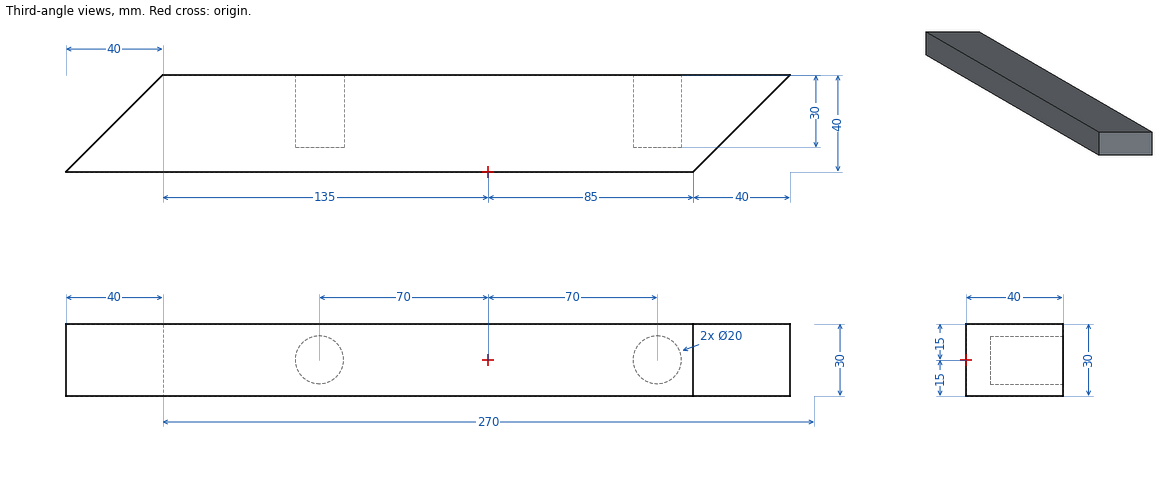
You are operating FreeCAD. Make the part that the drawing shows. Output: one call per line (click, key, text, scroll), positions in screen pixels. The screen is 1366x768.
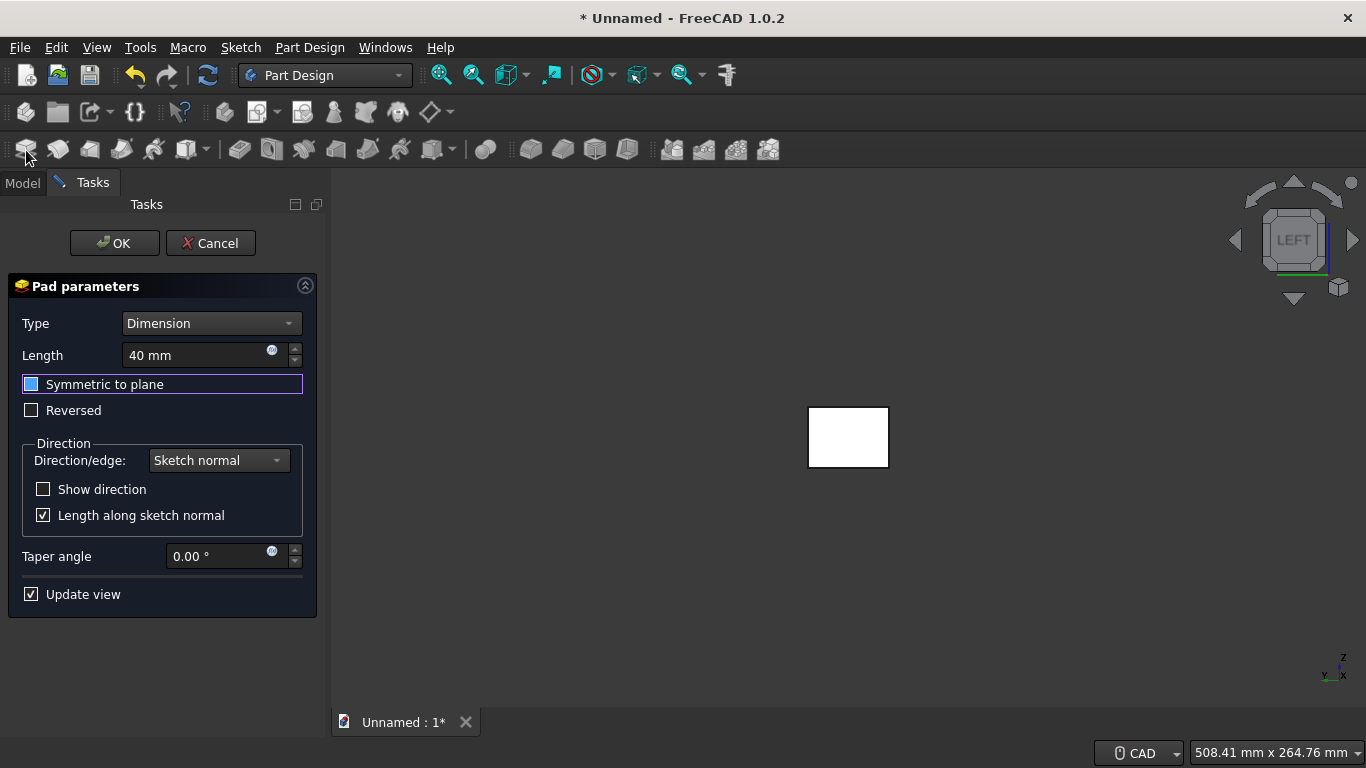
click(115, 243)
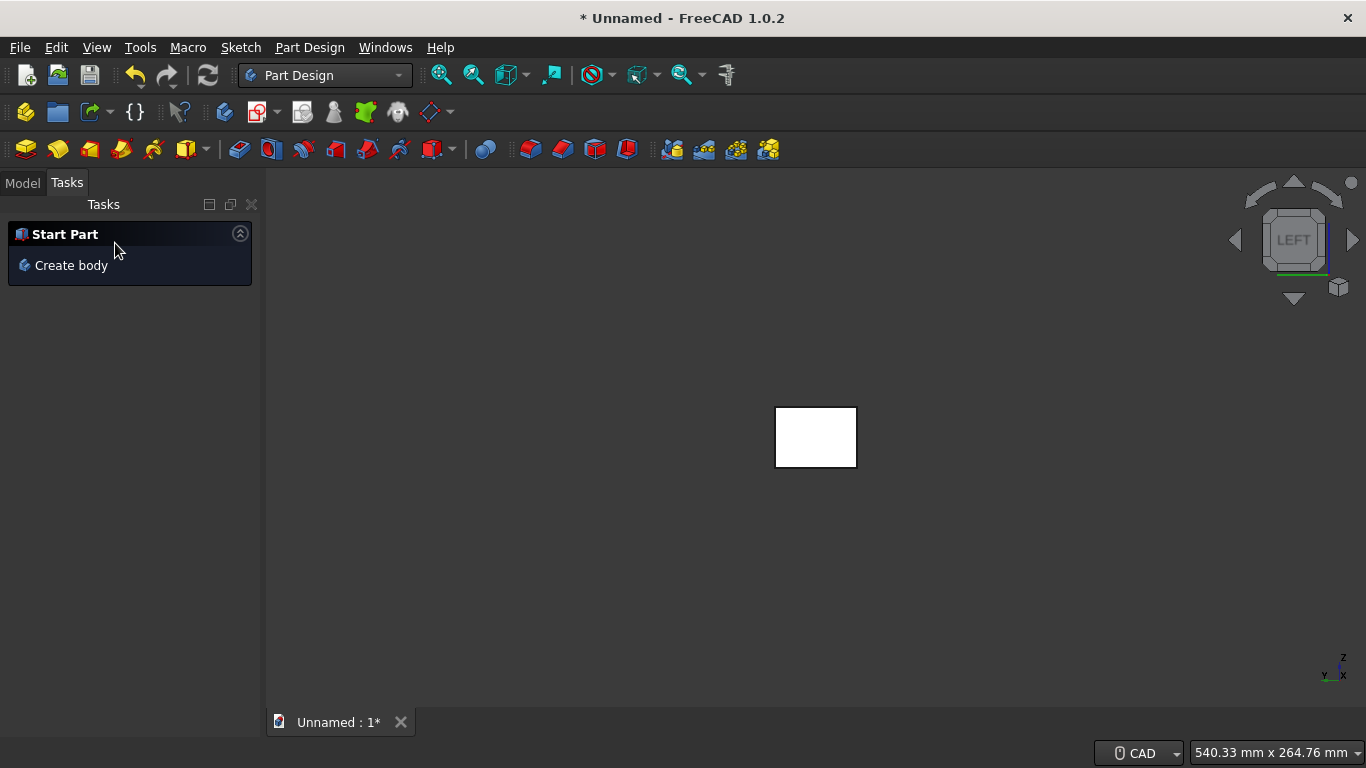
key(v)
key(f)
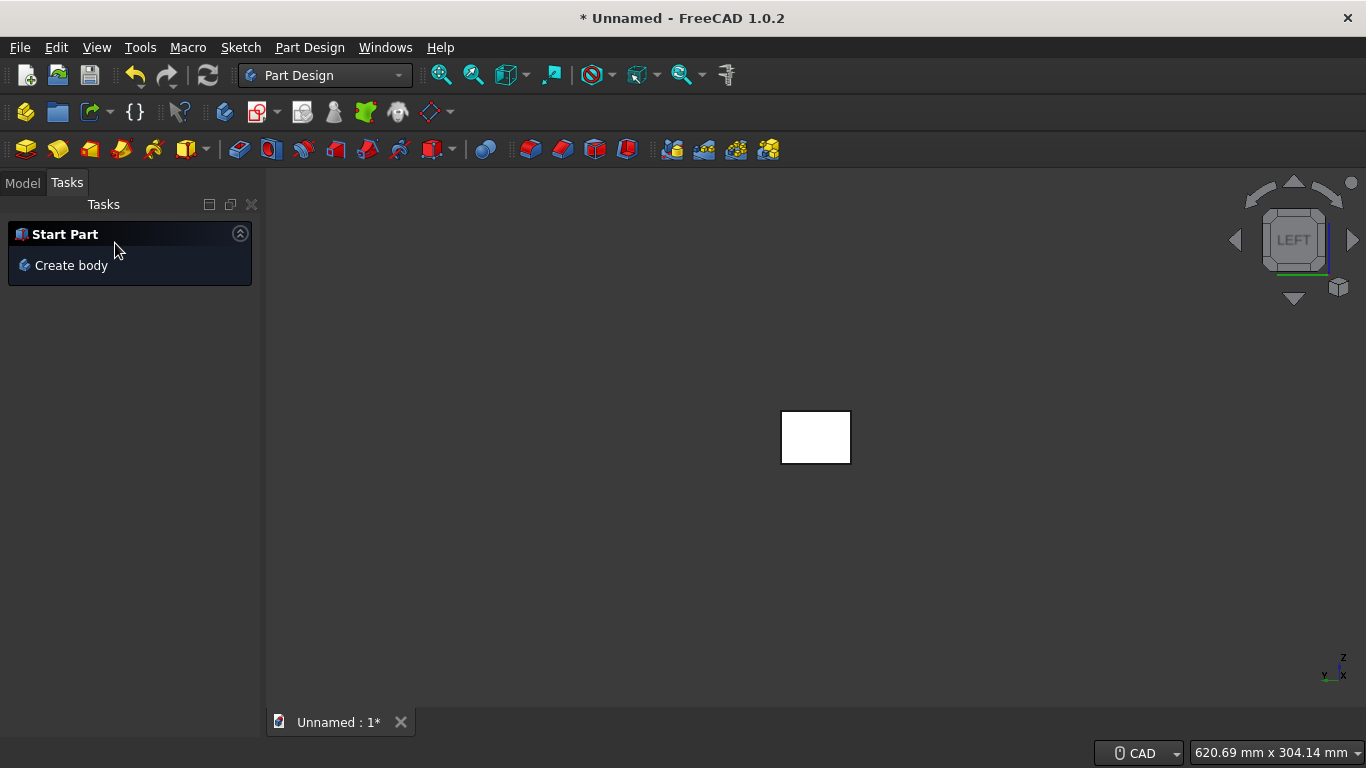
key(0)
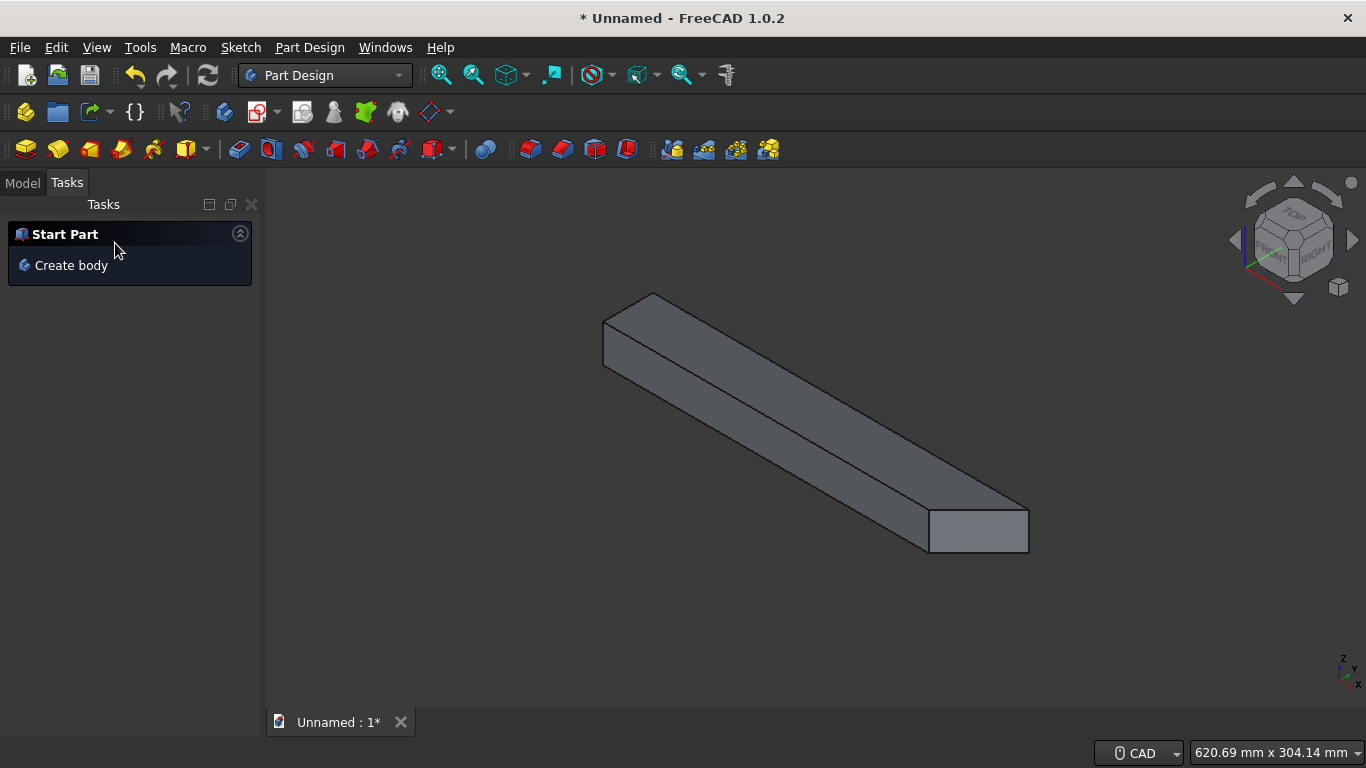
click(923, 477)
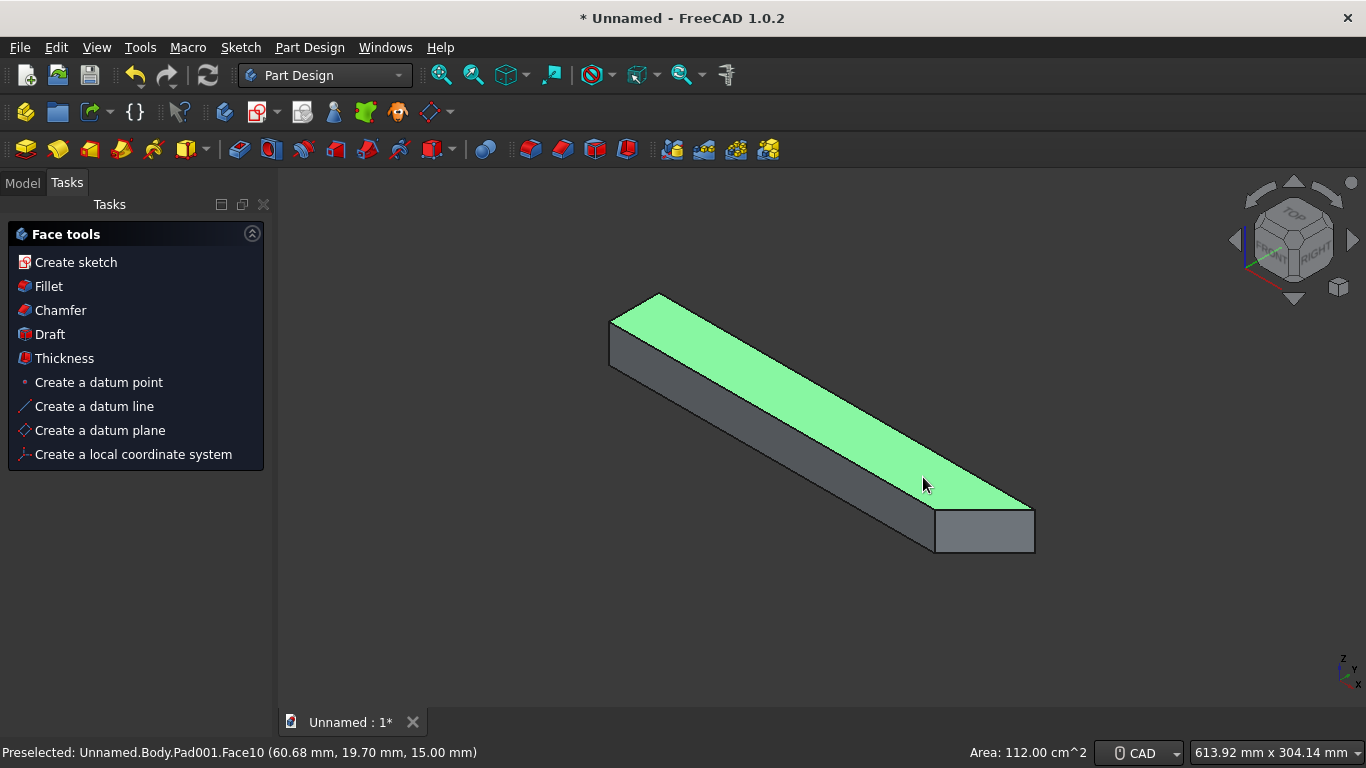
click(258, 112)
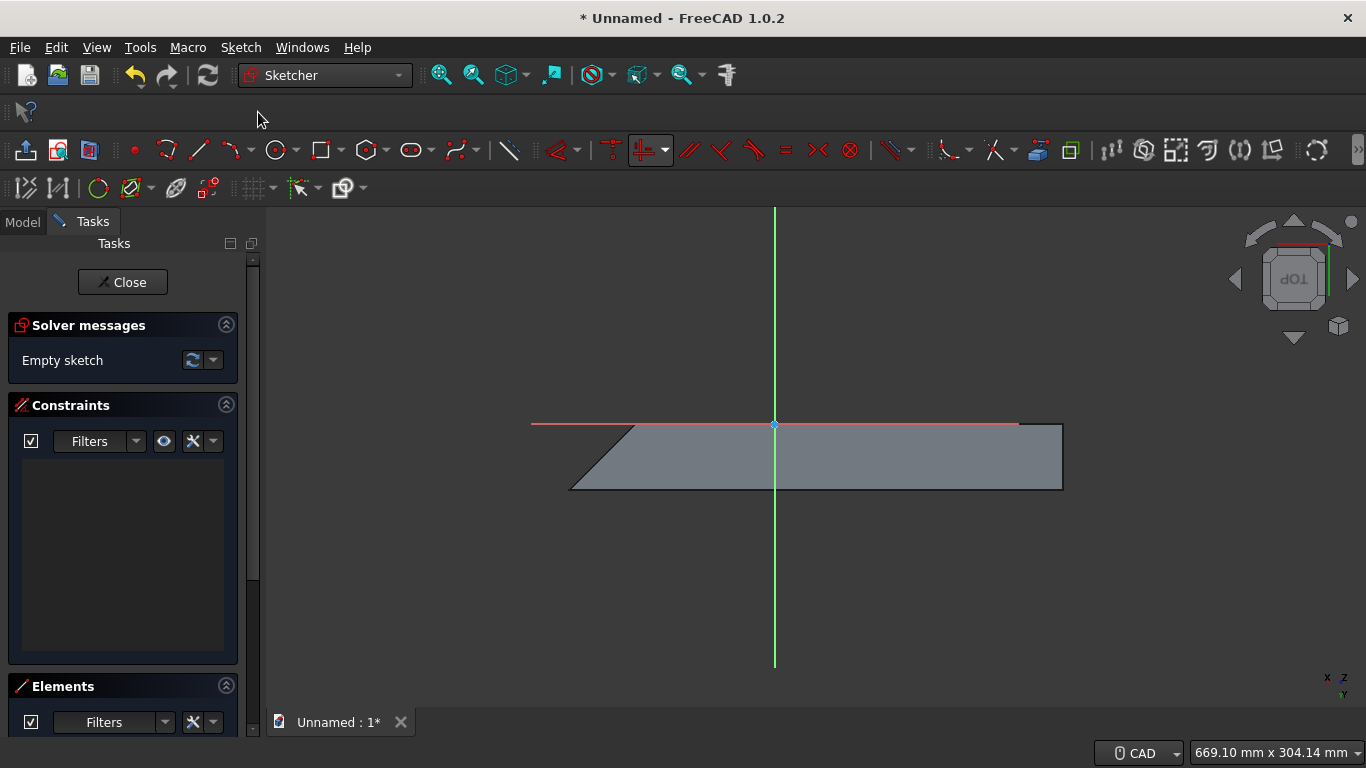
scroll(1101, 457, up, 8)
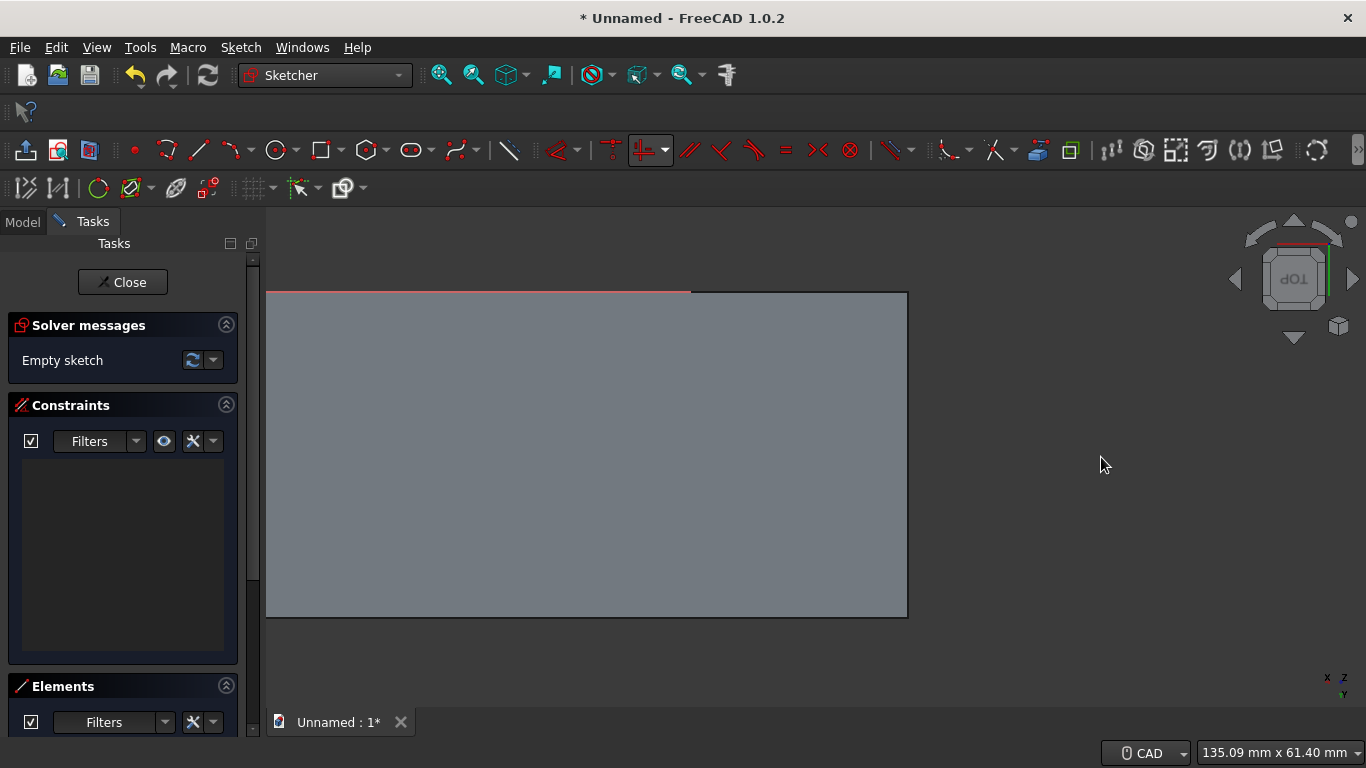
click(168, 150)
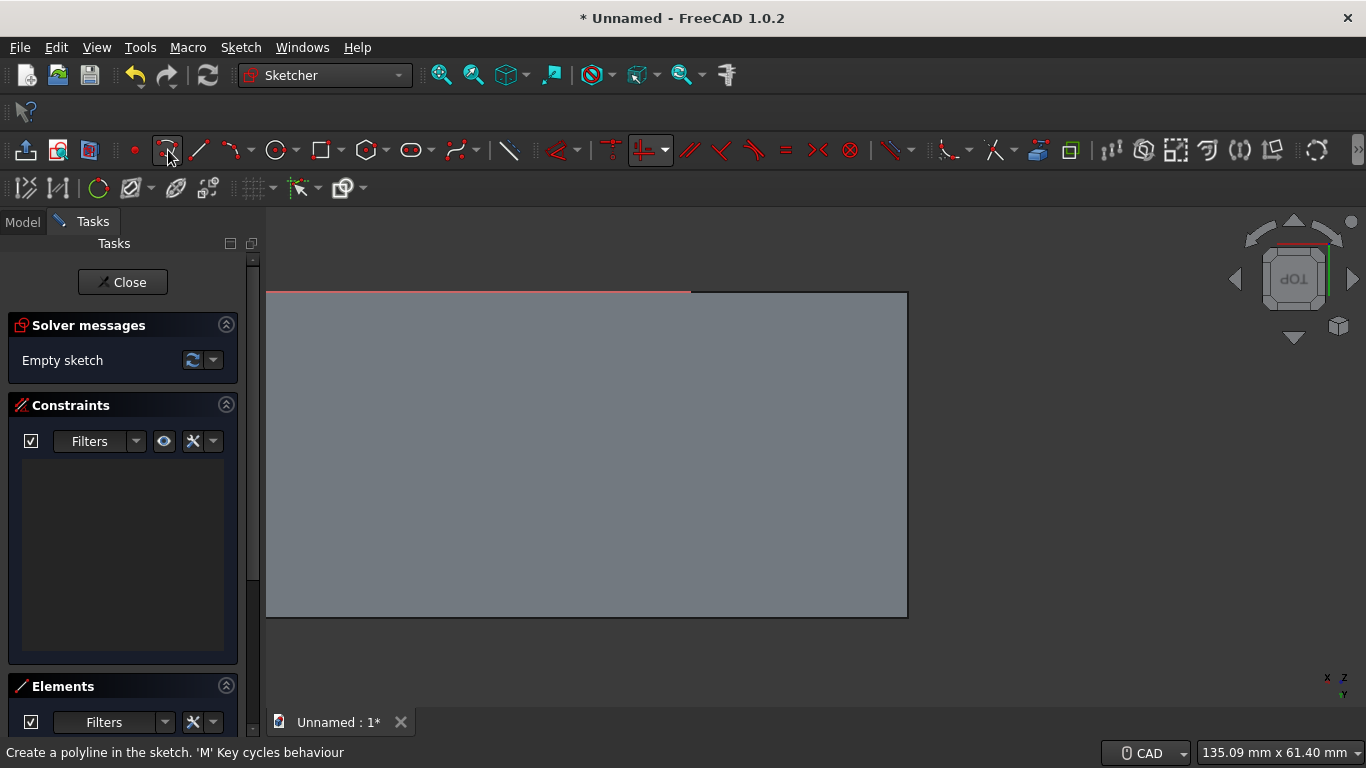
click(582, 618)
click(908, 618)
click(908, 292)
click(582, 619)
key(Escape)
key(Escape)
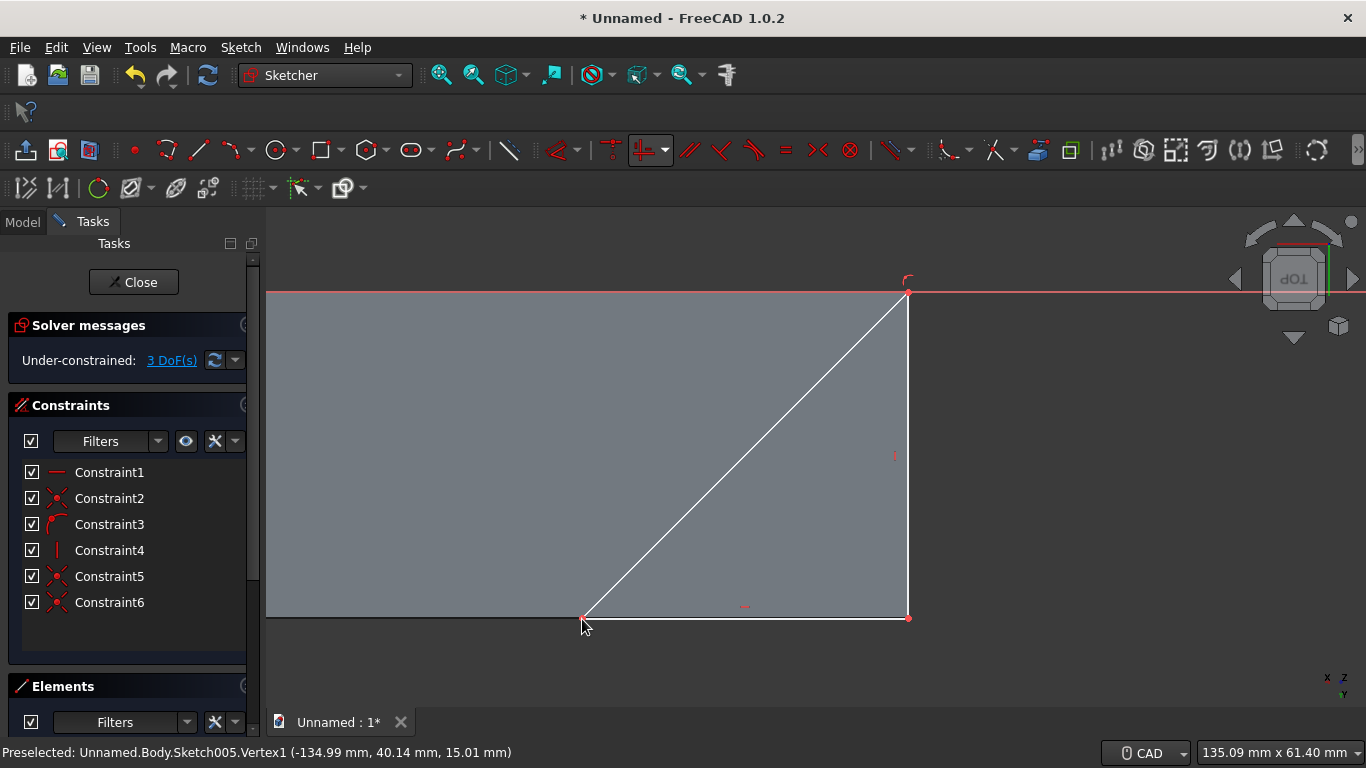
click(556, 150)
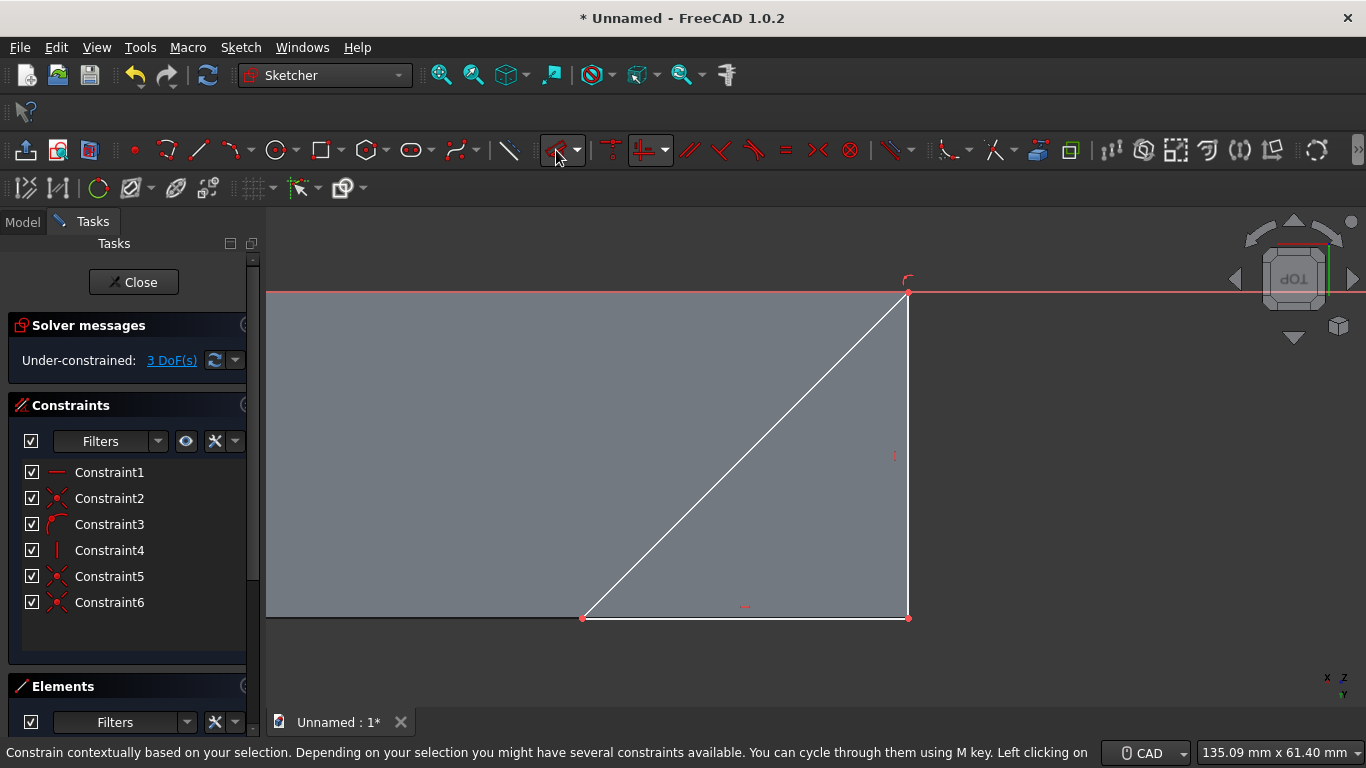
click(680, 619)
click(745, 653)